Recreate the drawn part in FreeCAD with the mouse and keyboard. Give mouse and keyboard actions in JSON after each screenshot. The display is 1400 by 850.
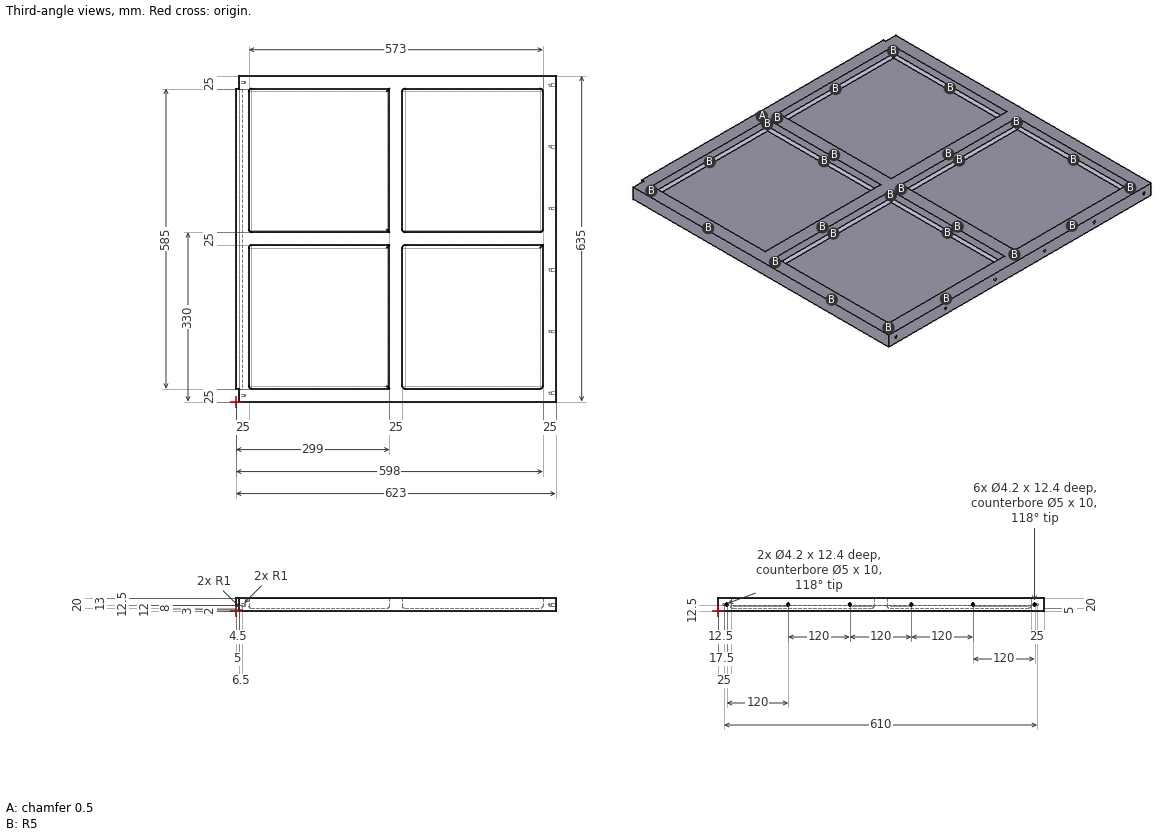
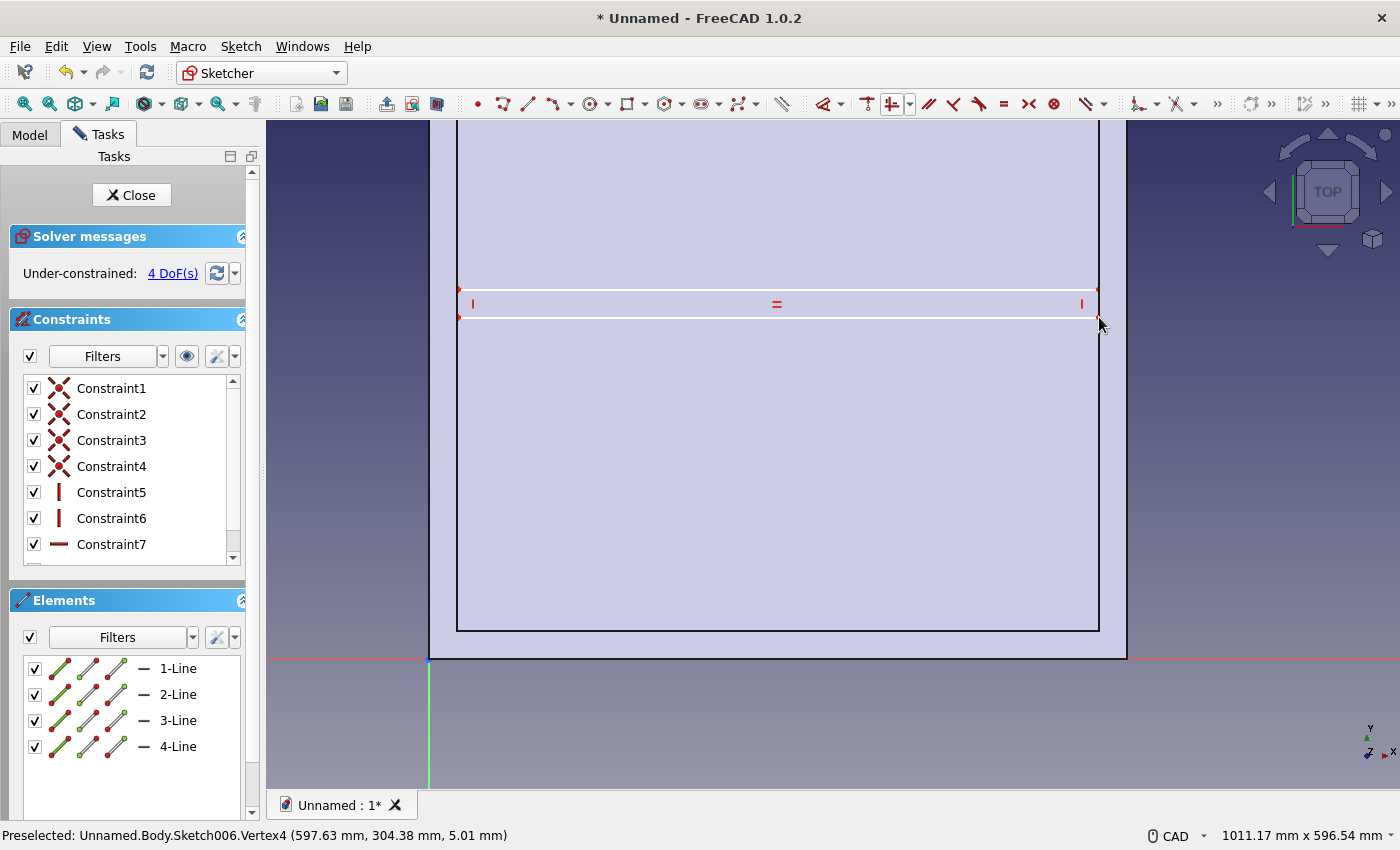
{"action": "left_click", "coordinate": [822, 104]}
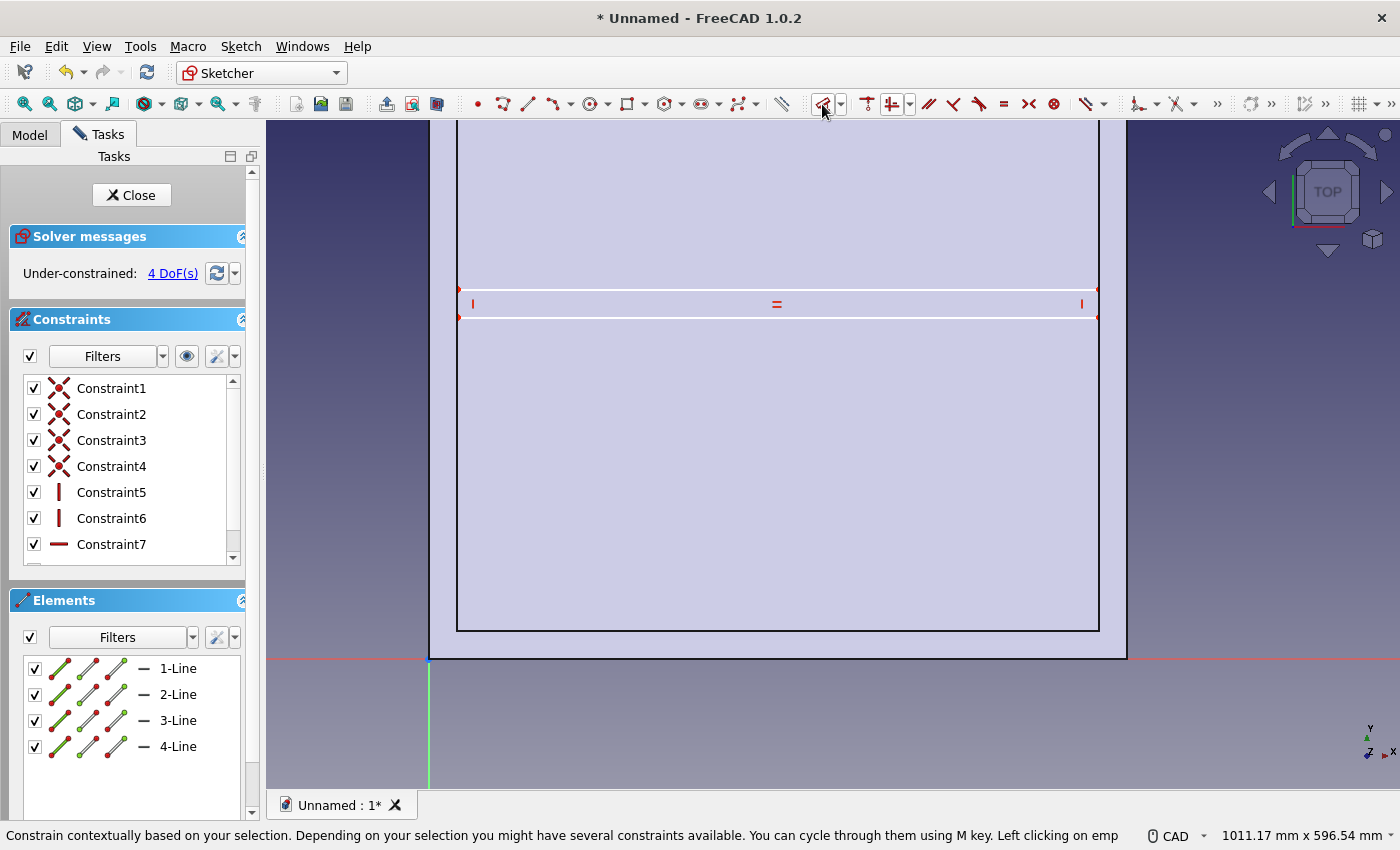
{"action": "scroll", "coordinate": [457, 301], "scroll_direction": "up", "scroll_amount": 2}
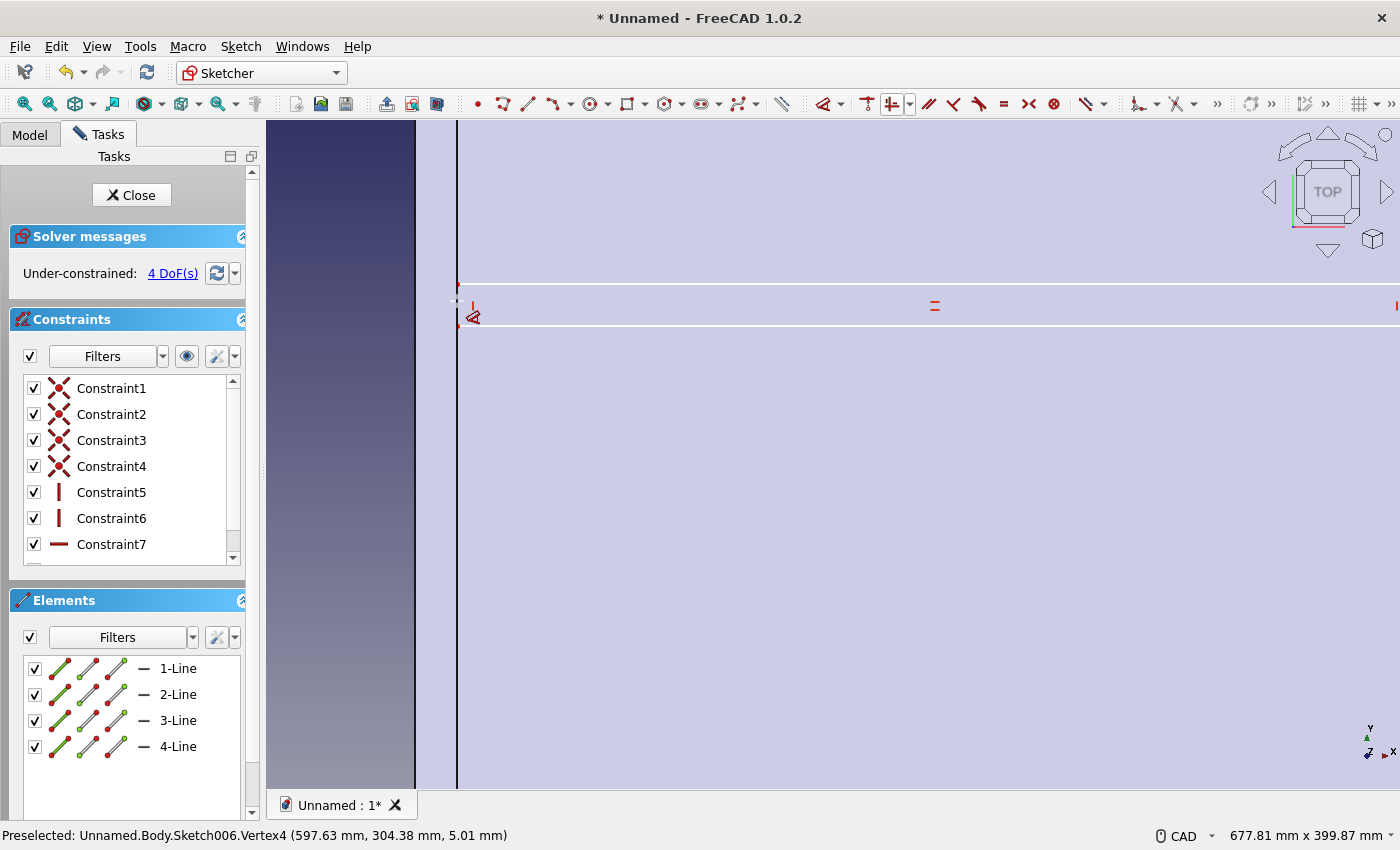
{"action": "left_click", "coordinate": [457, 301]}
{"action": "left_click", "coordinate": [491, 305]}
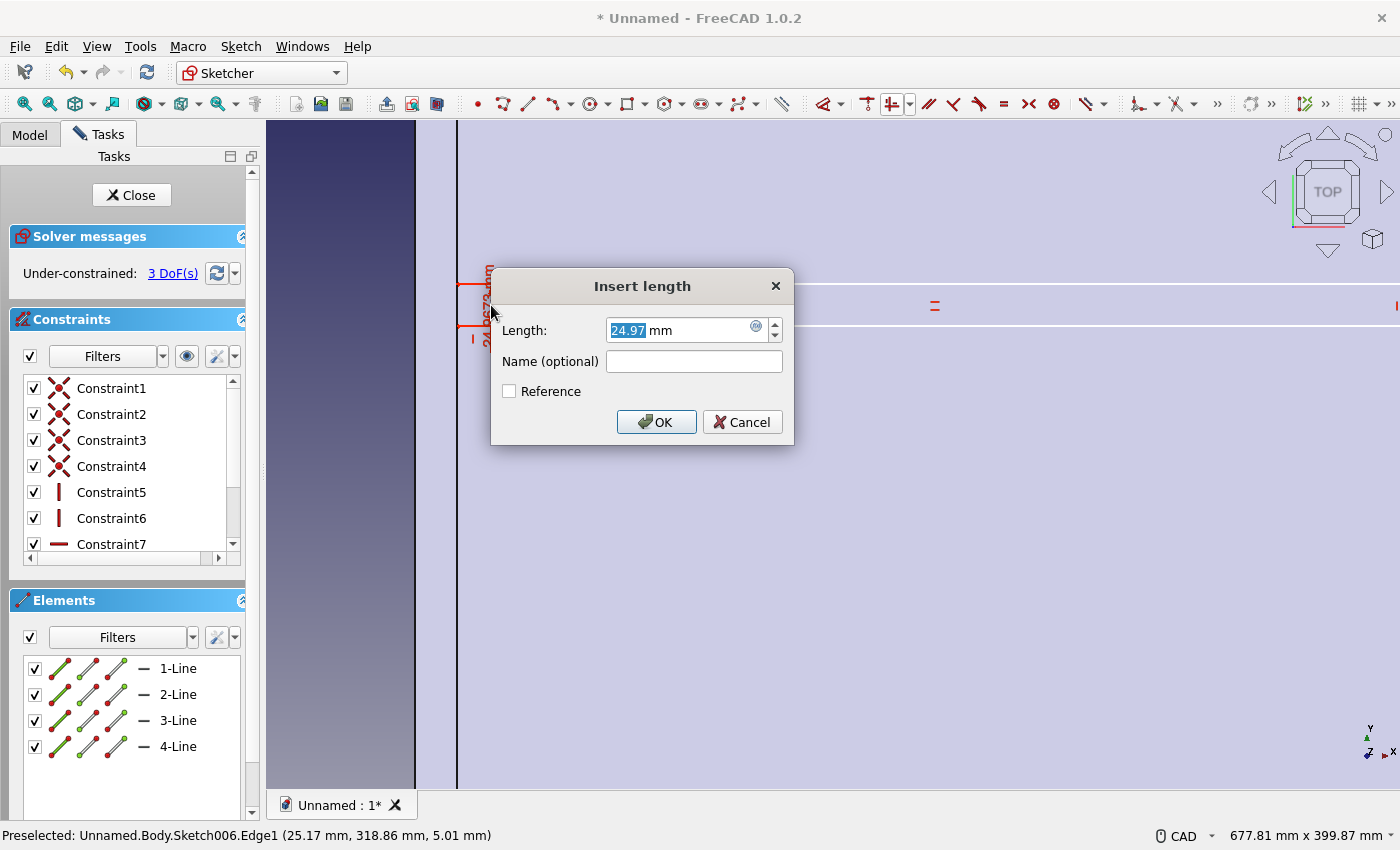
{"action": "type", "text": "25"}
{"action": "key", "text": "Return"}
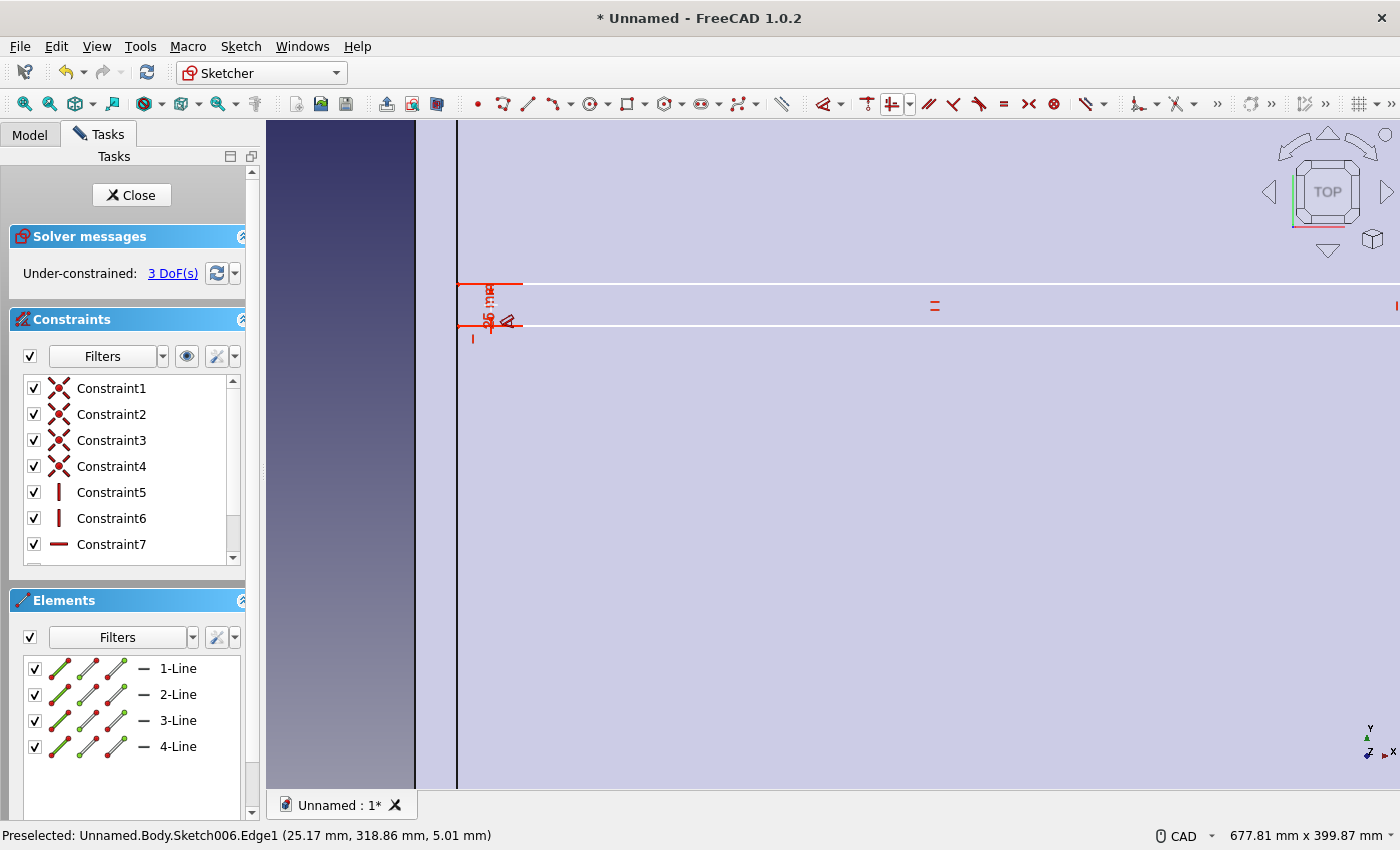
{"action": "left_click", "coordinate": [744, 326]}
{"action": "left_click", "coordinate": [846, 360]}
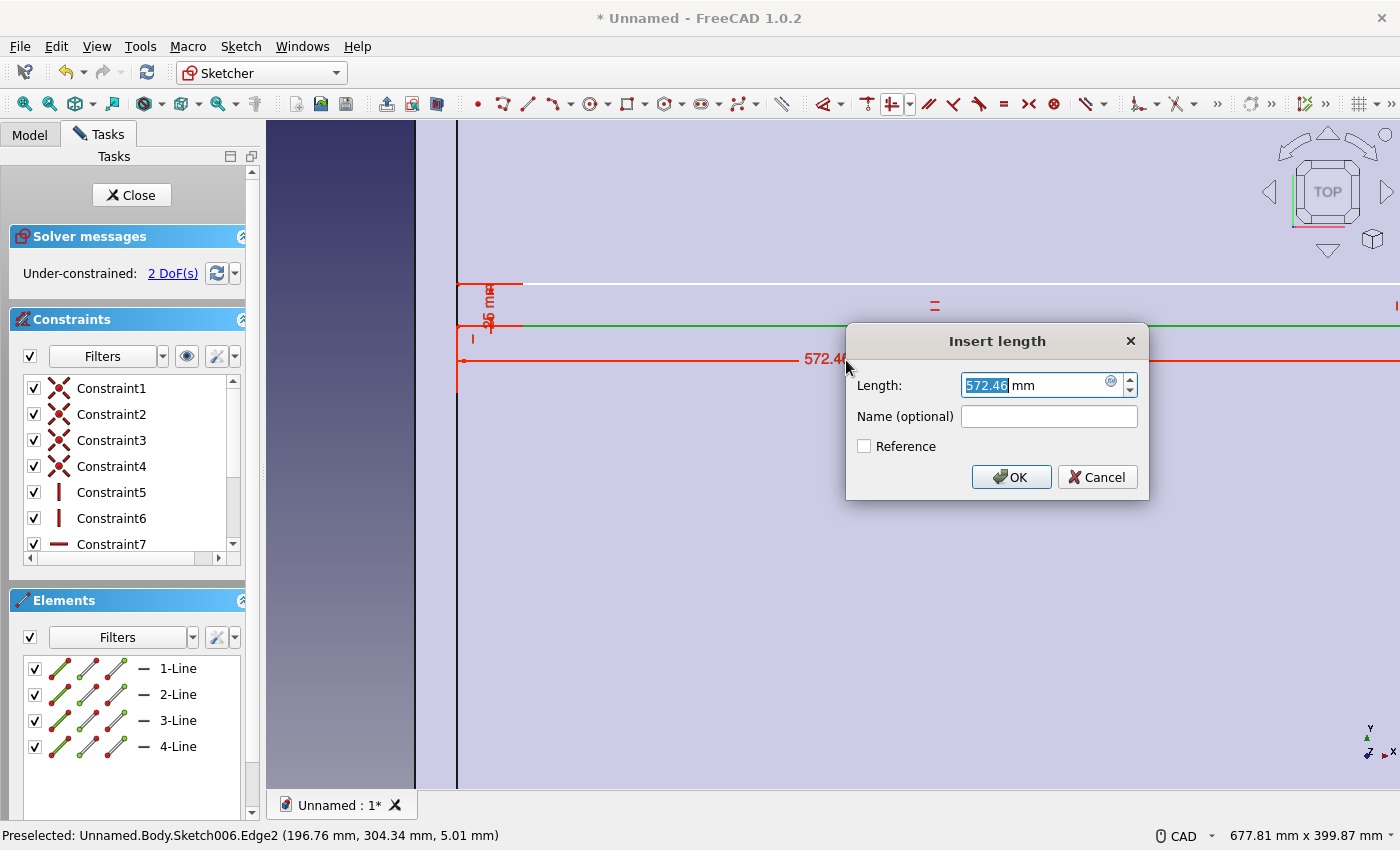
{"action": "type", "text": "573"}
{"action": "key", "text": "Return"}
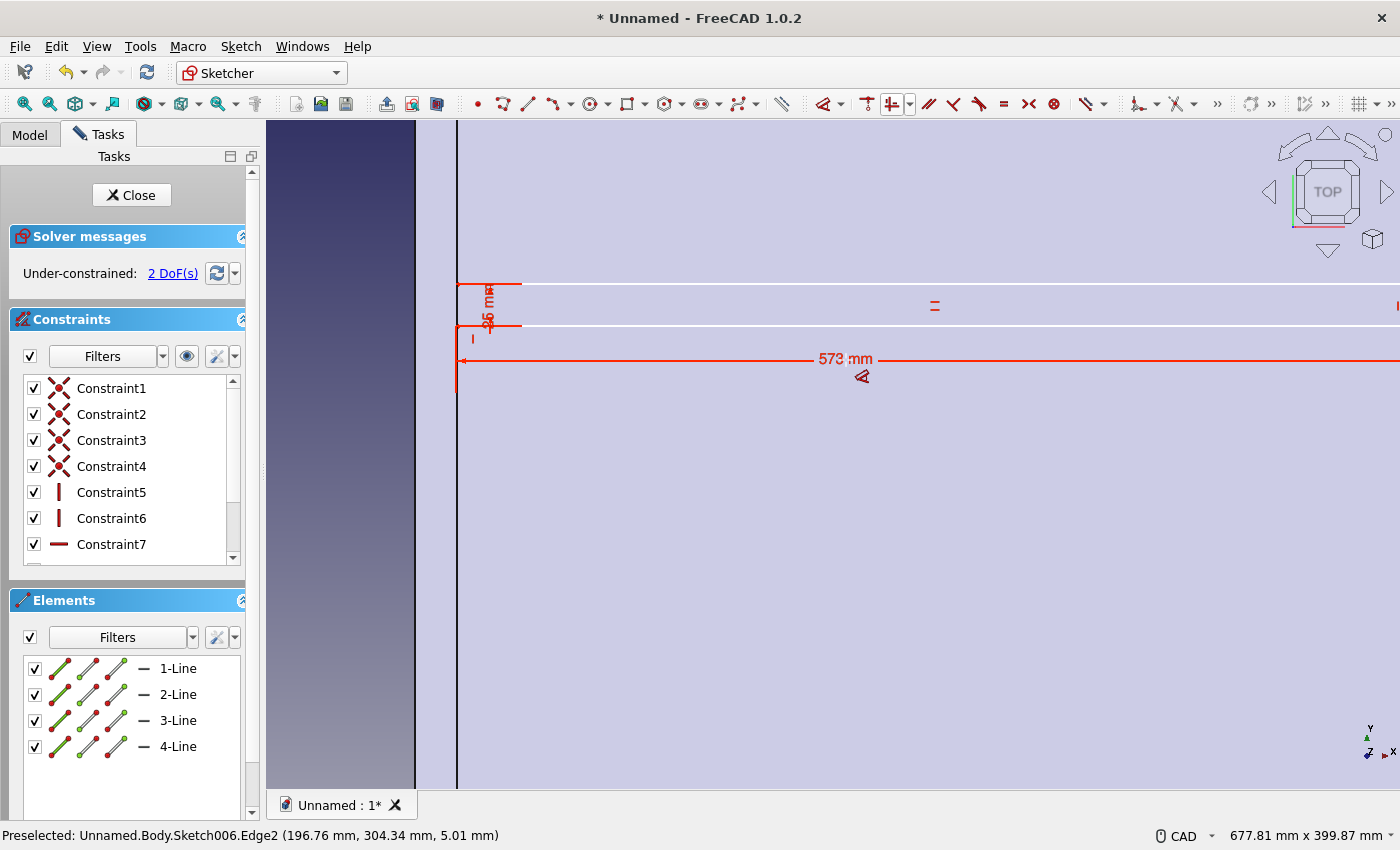
{"action": "left_click", "coordinate": [456, 284]}
{"action": "left_click", "coordinate": [436, 250]}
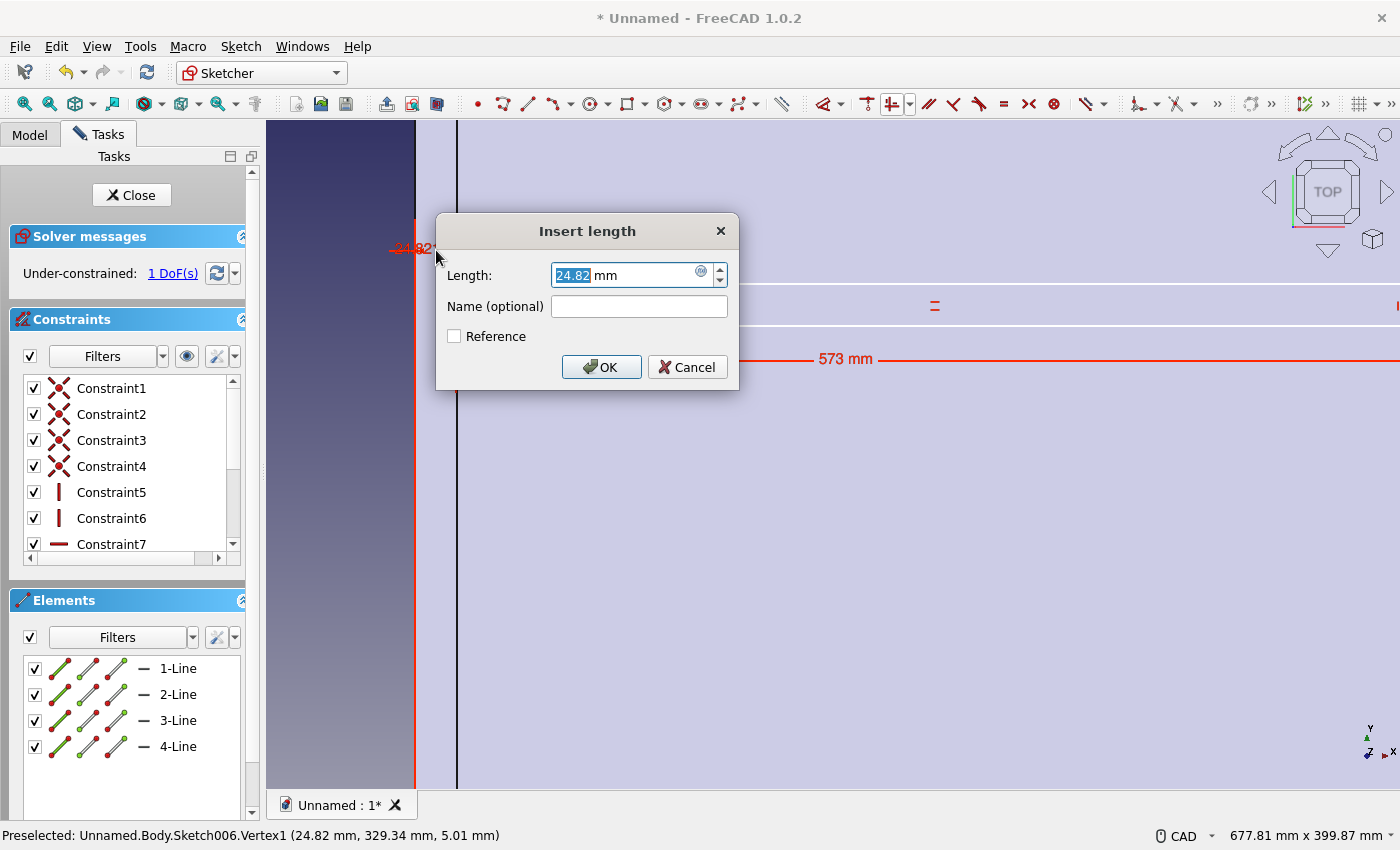
{"action": "type", "text": "25"}
{"action": "key", "text": "Return"}